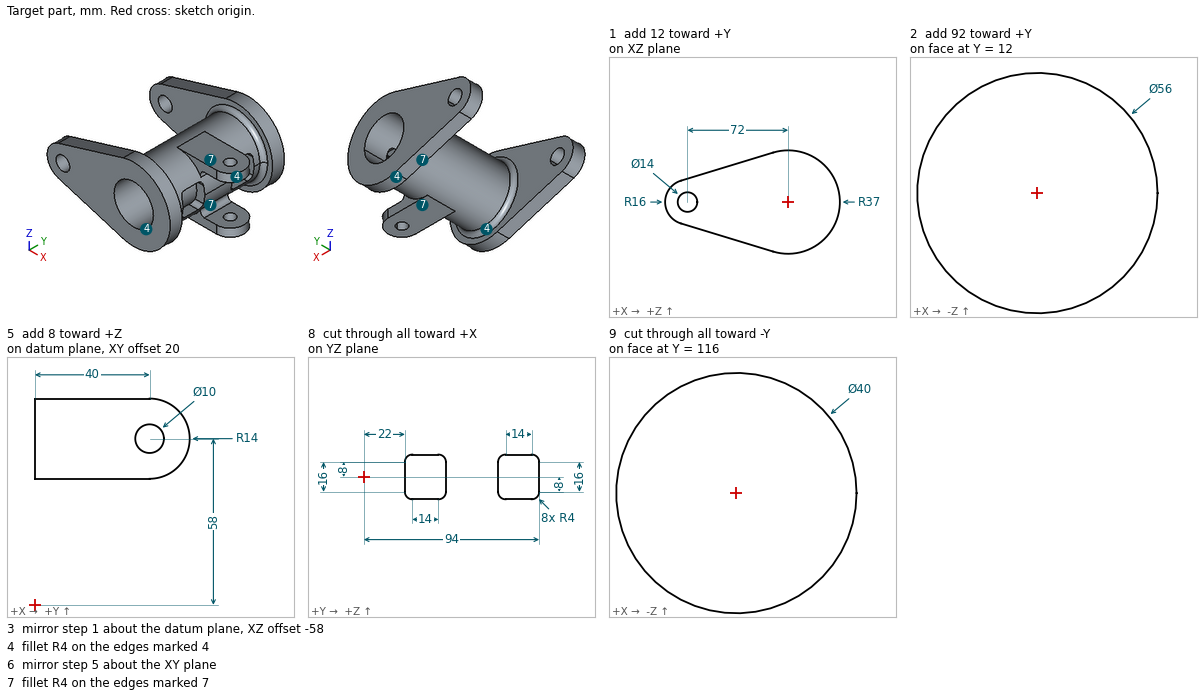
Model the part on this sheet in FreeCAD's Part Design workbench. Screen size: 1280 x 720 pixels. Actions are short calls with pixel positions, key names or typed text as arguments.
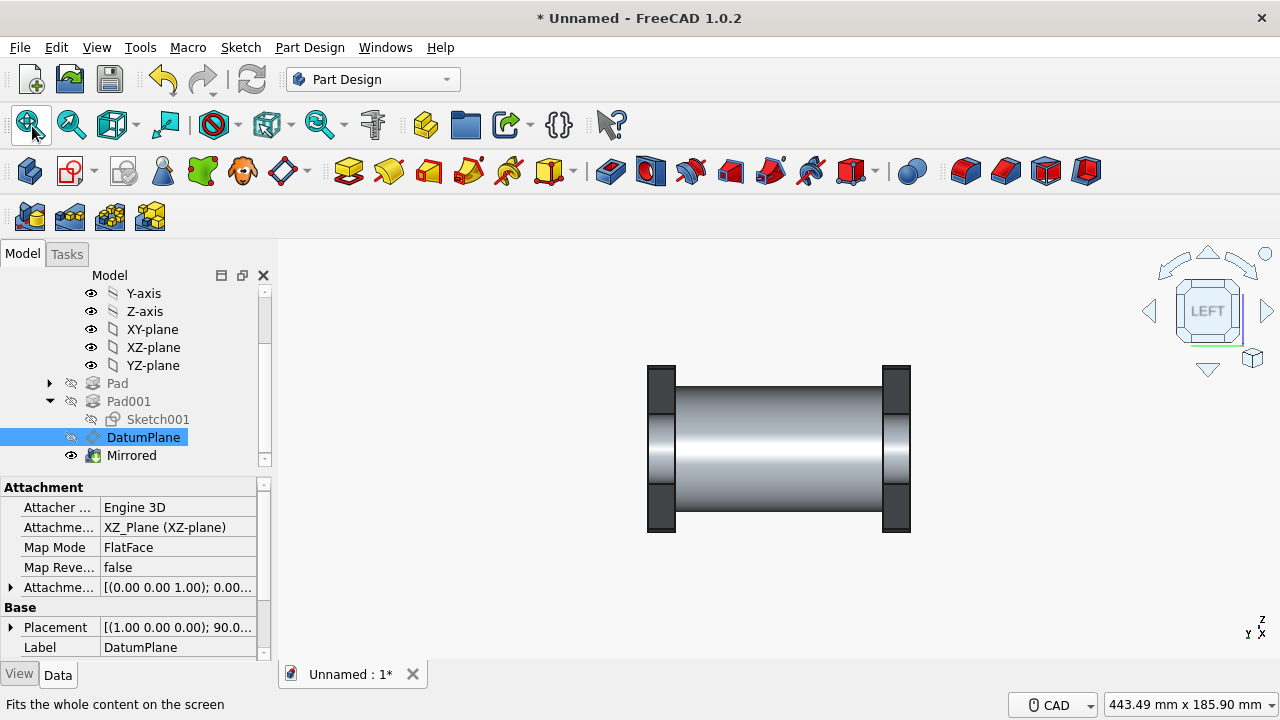
key(v)
key(3)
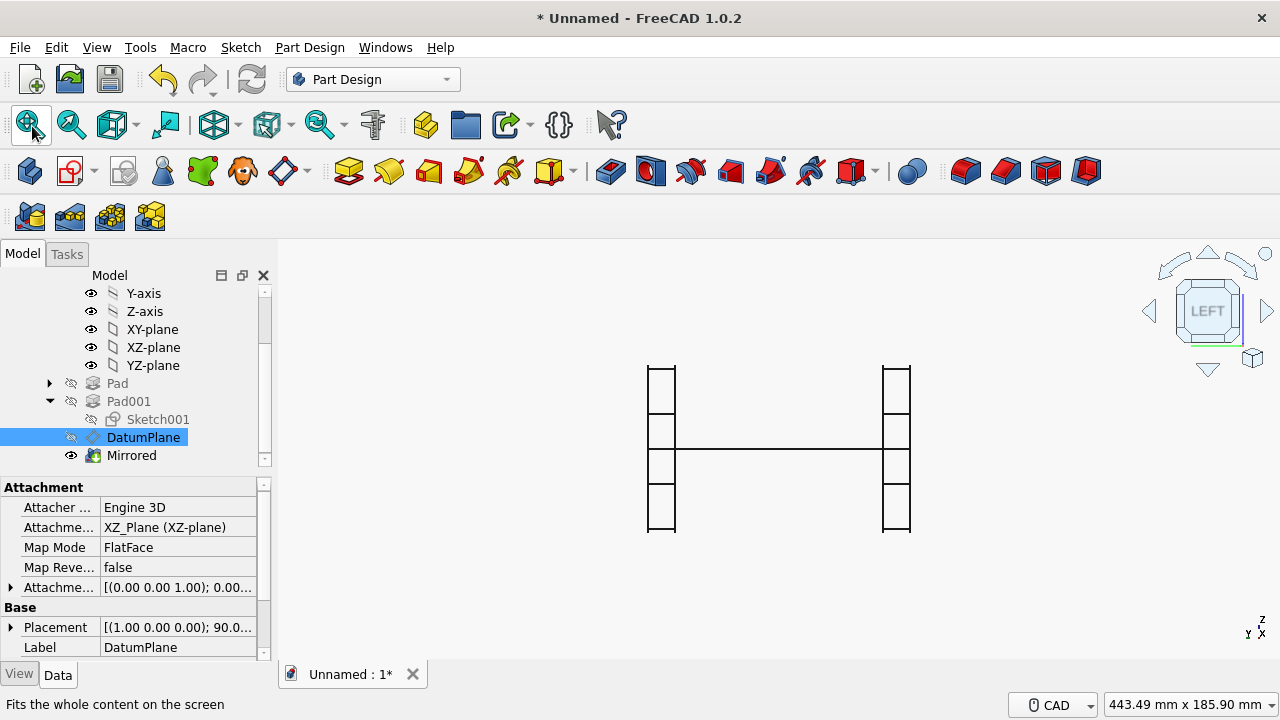
key(0)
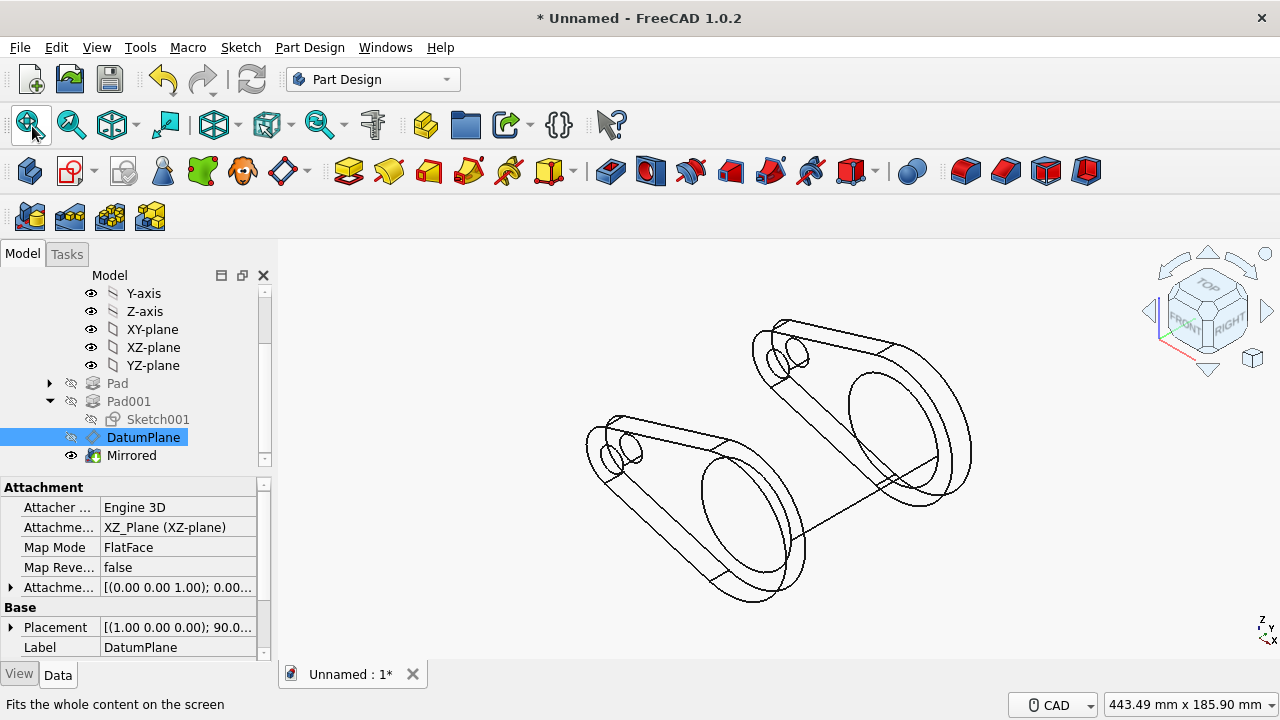
click(702, 488)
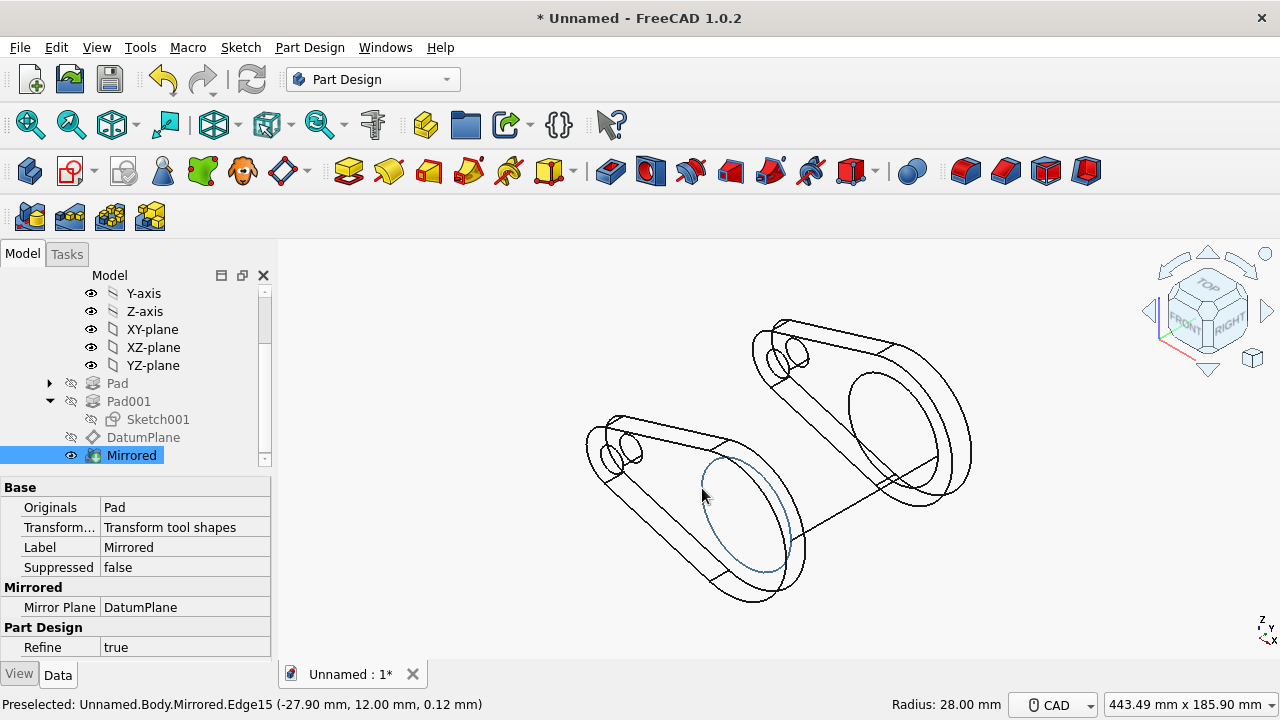
click(848, 403, ctrl)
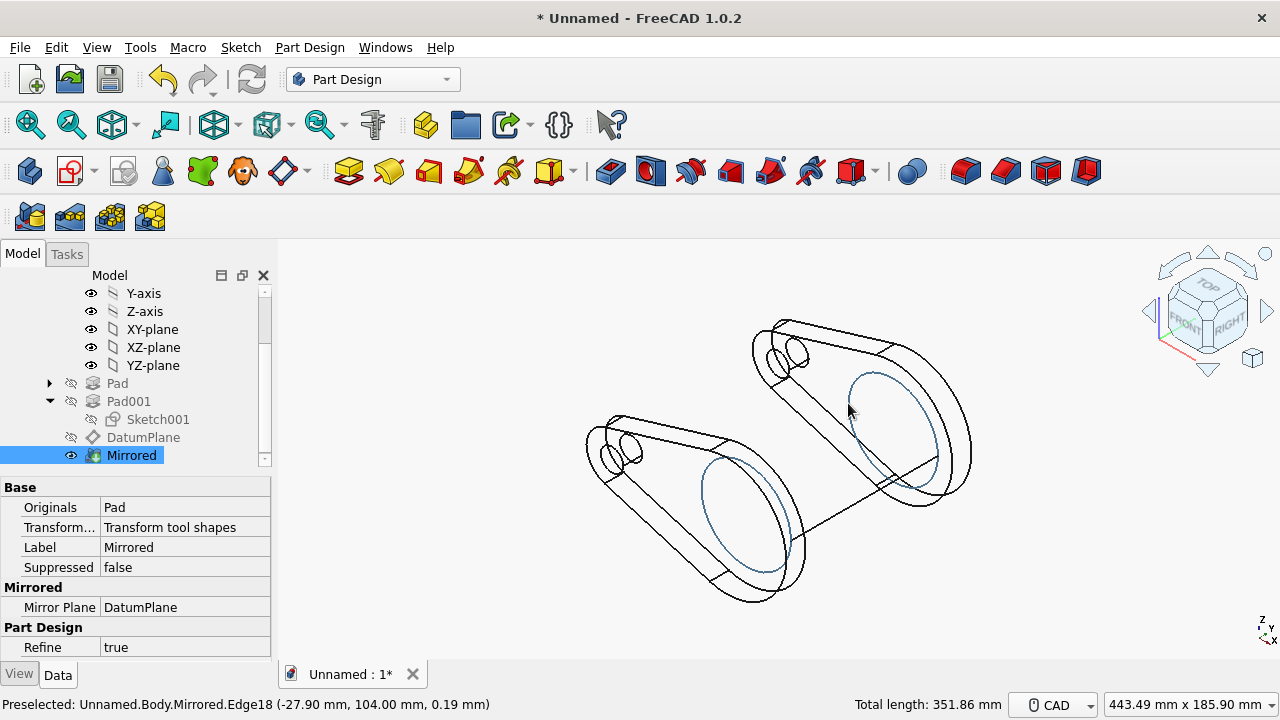
key(v)
key(1)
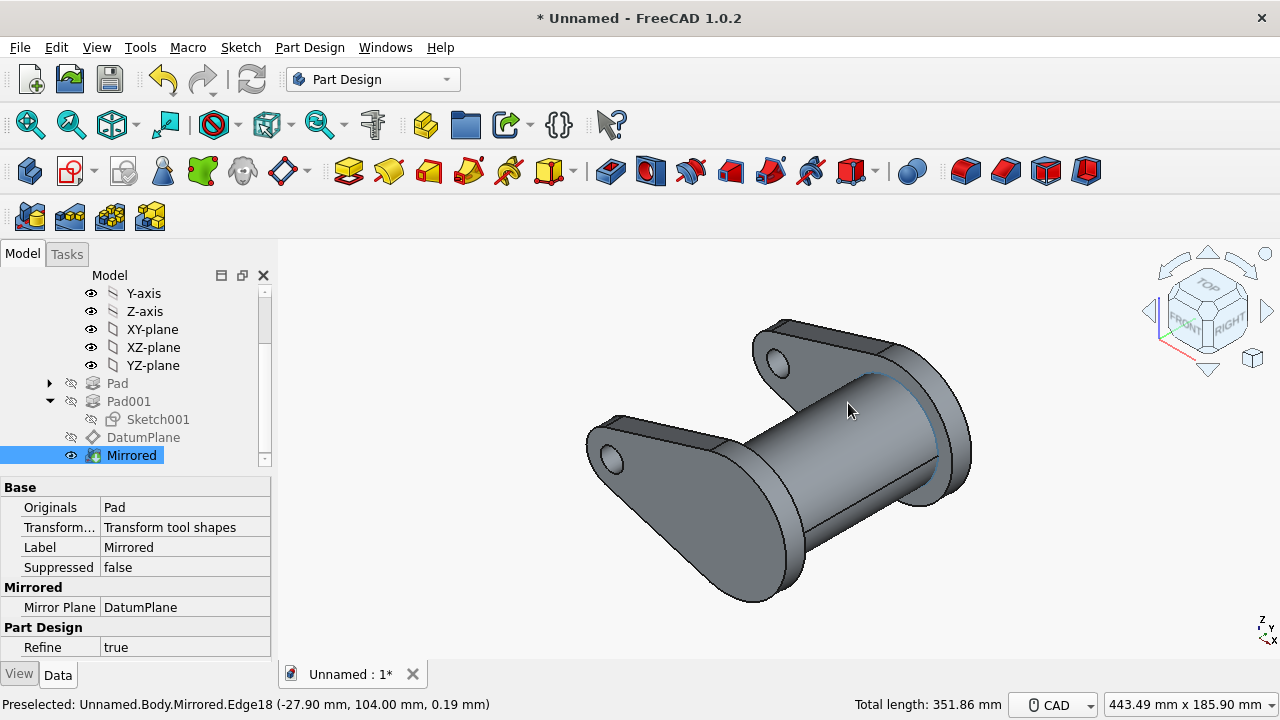
click(966, 172)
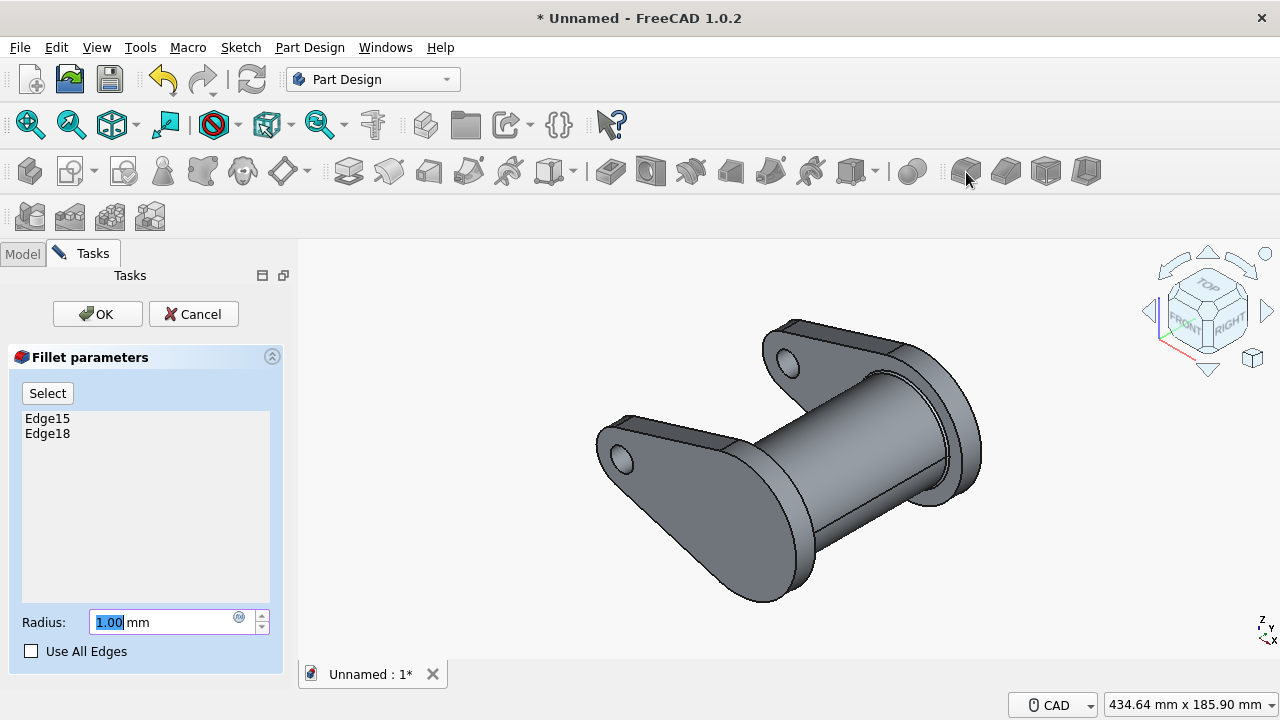
text(4)
key(Tab)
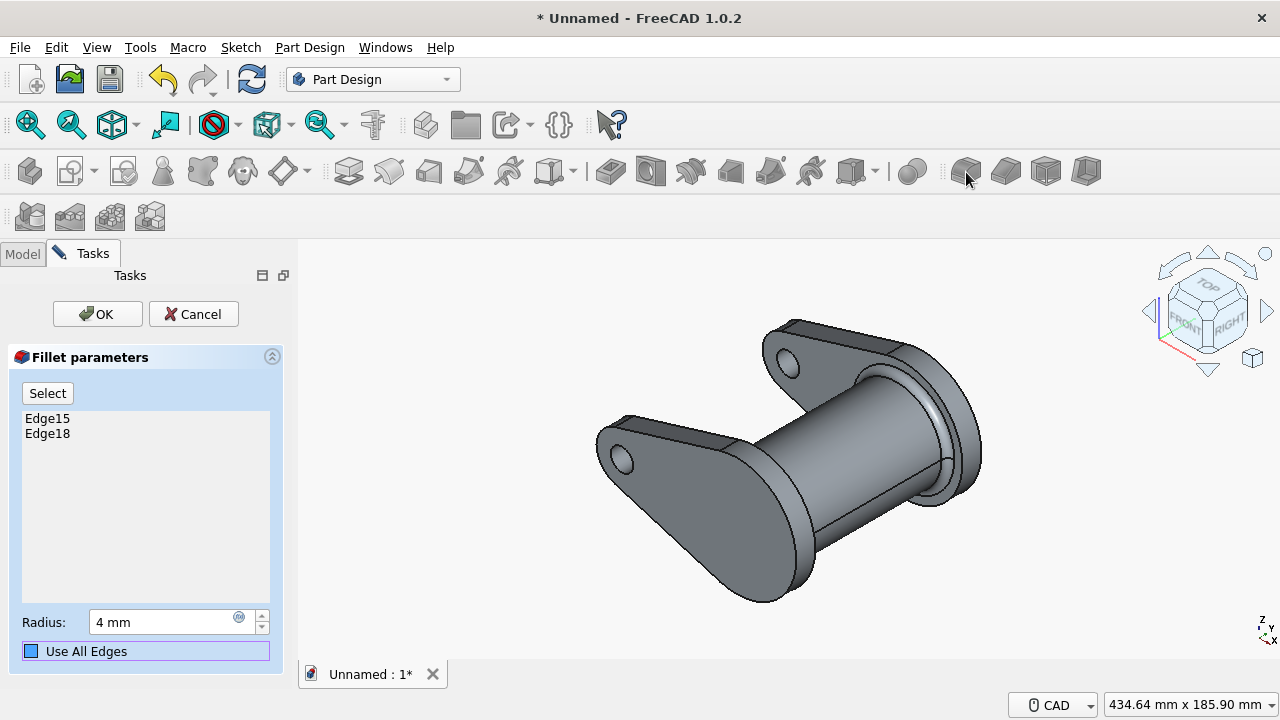
click(98, 314)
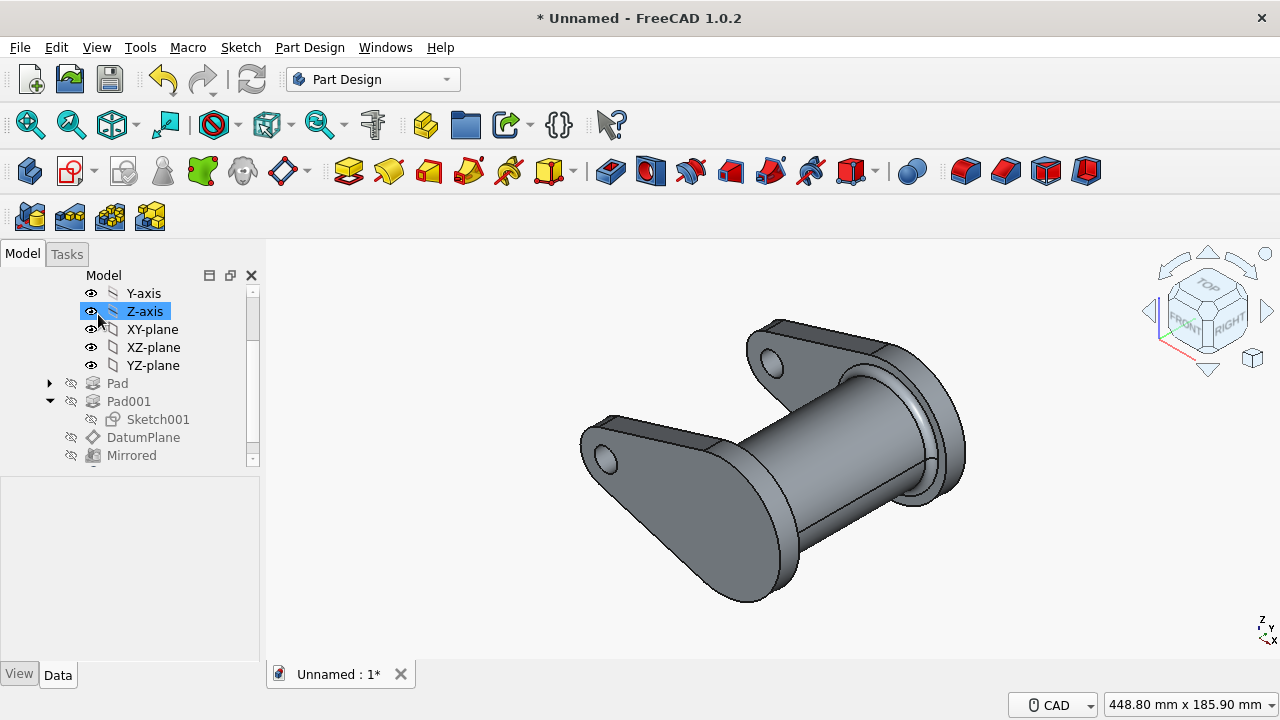
scroll(160, 379, down, 3)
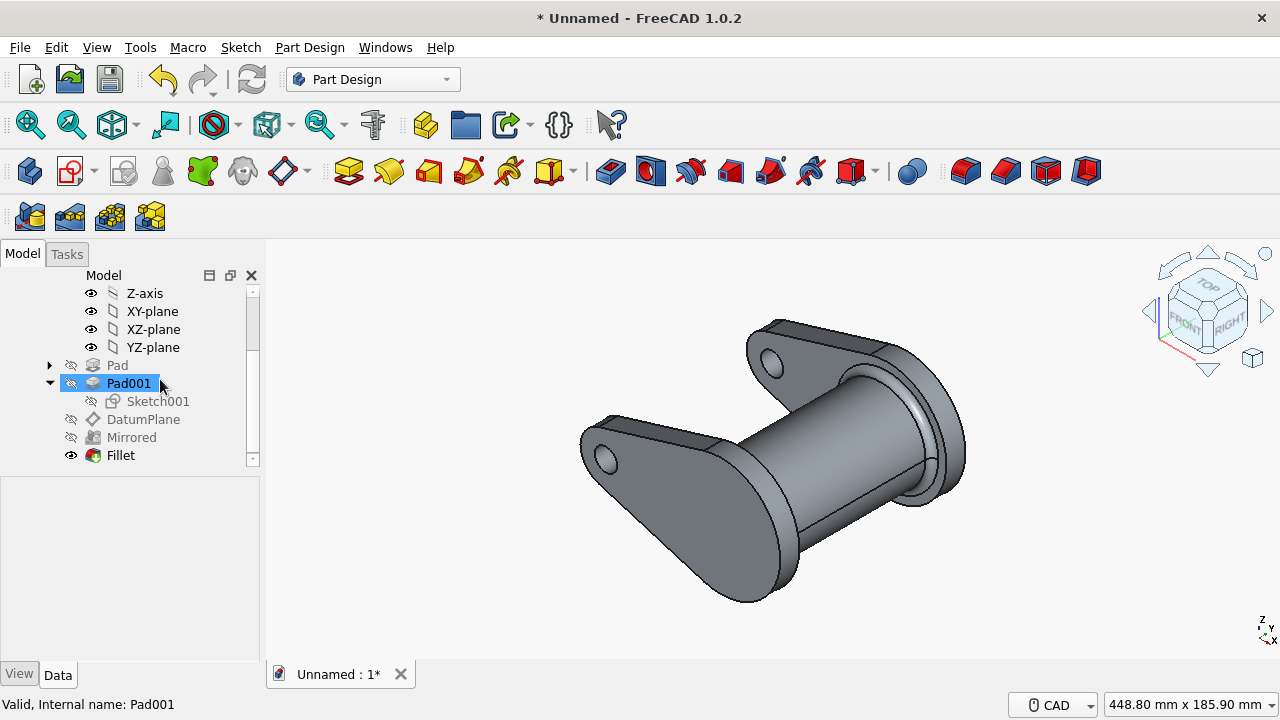
scroll(160, 379, up, 15)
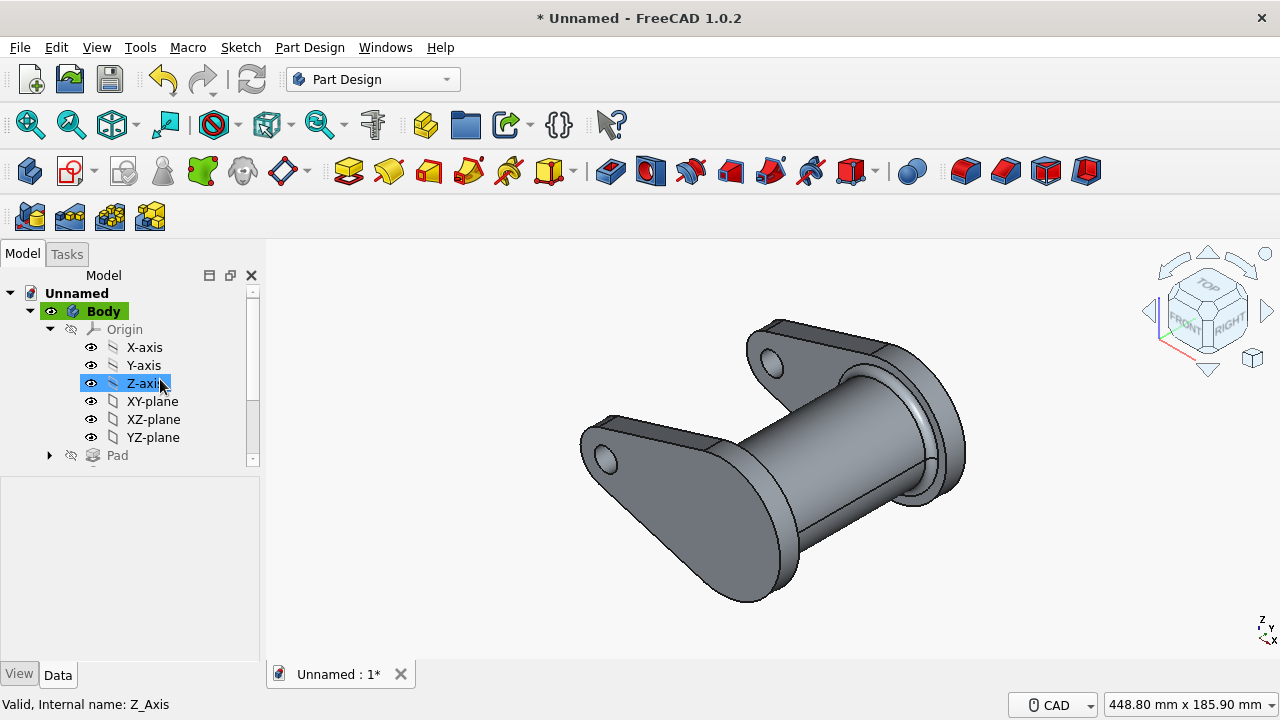
click(136, 401)